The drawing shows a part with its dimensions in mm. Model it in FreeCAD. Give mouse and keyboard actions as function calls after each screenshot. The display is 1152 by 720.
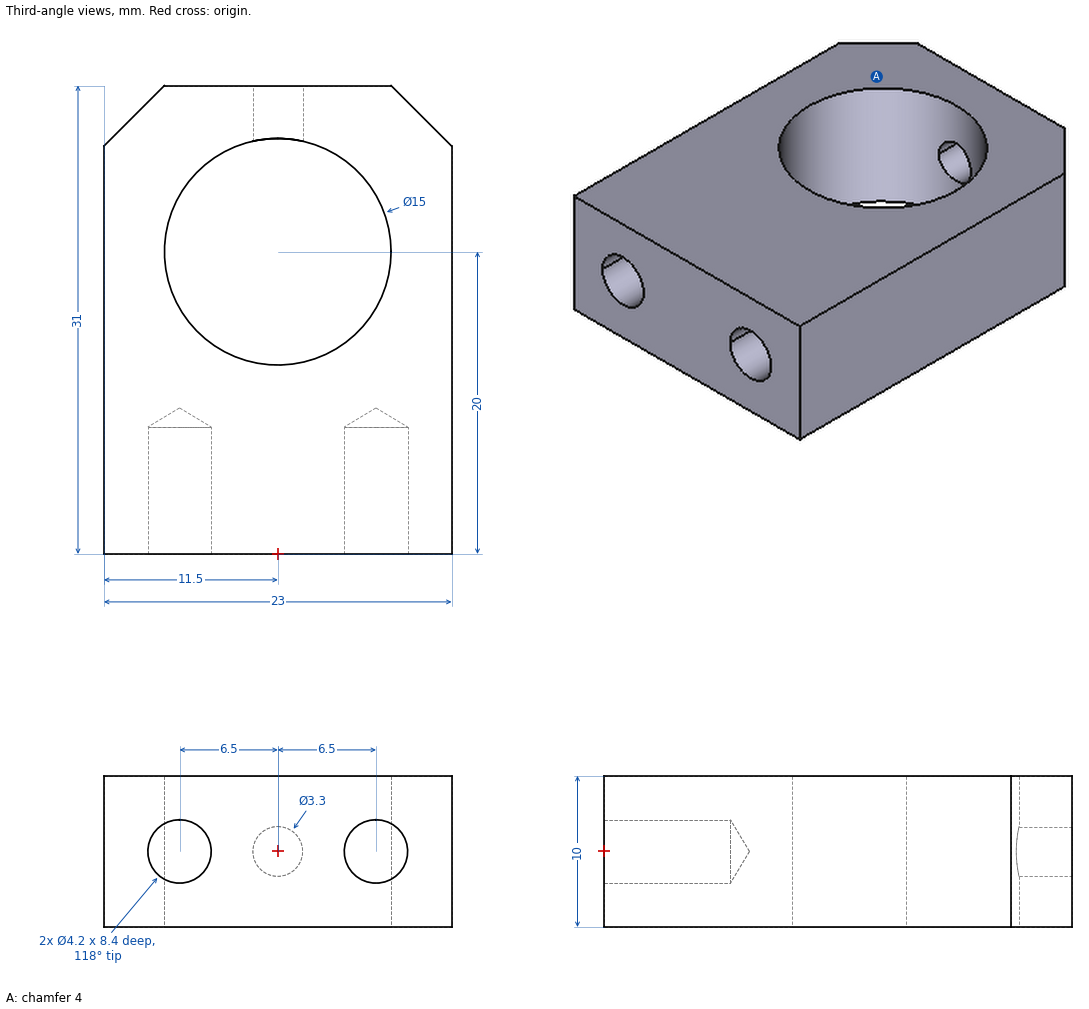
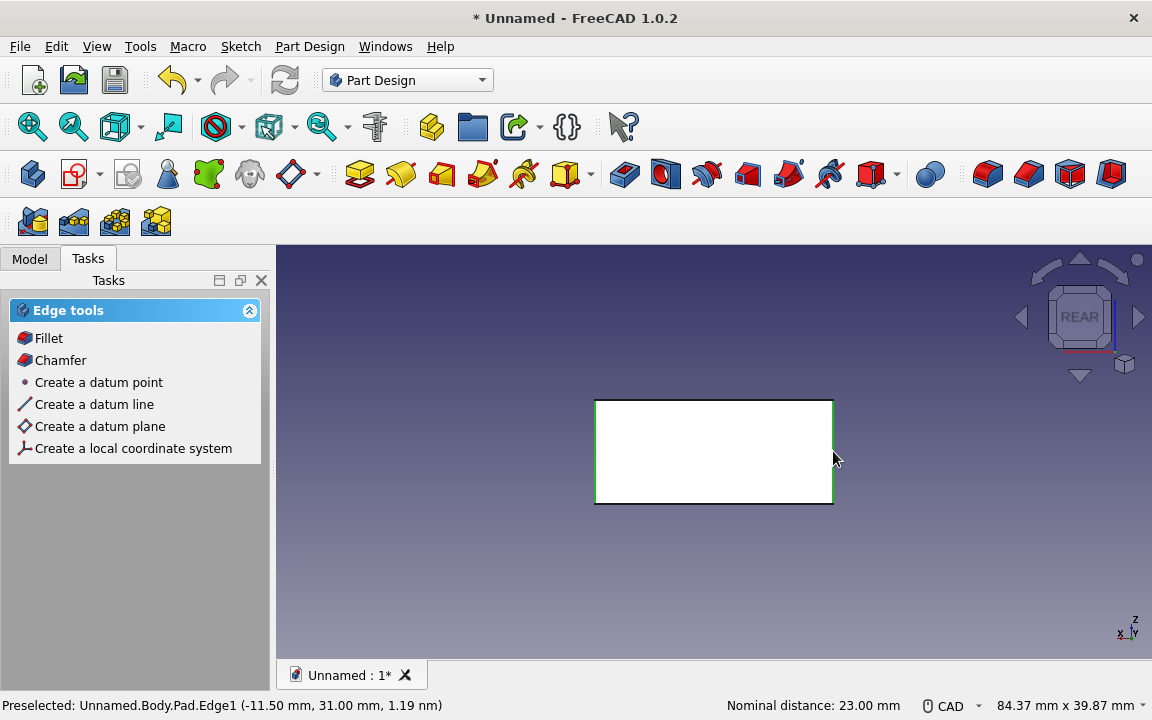
click(1029, 174)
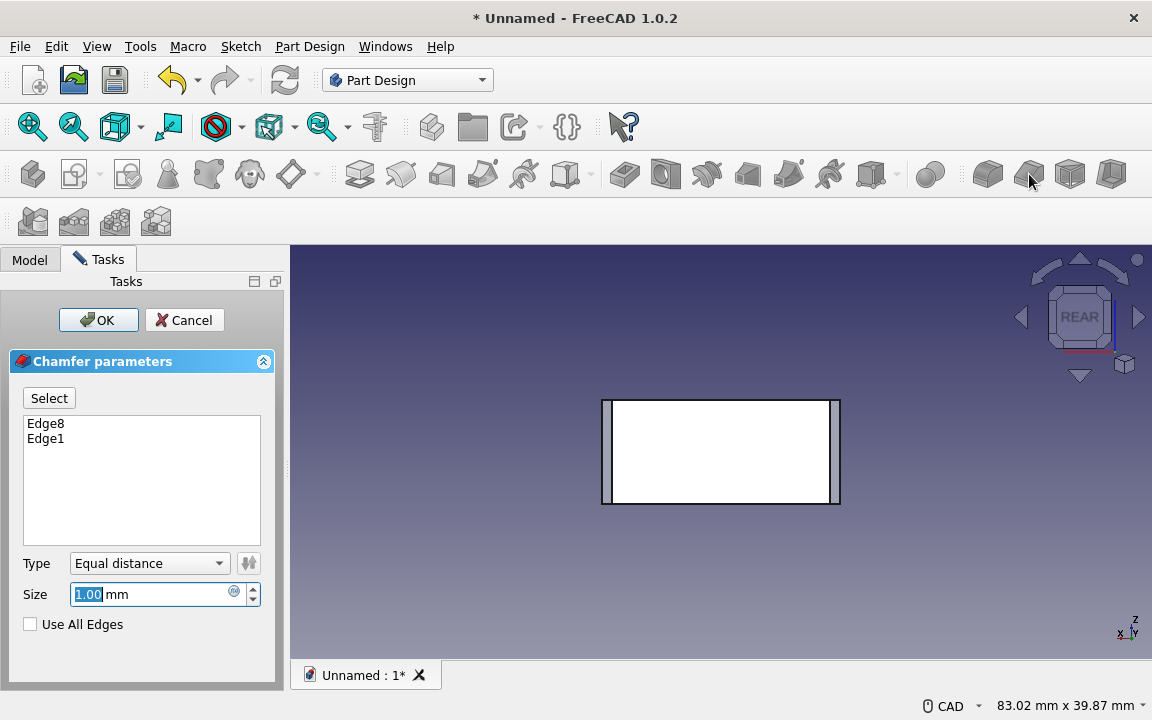
text(4)
key(Tab)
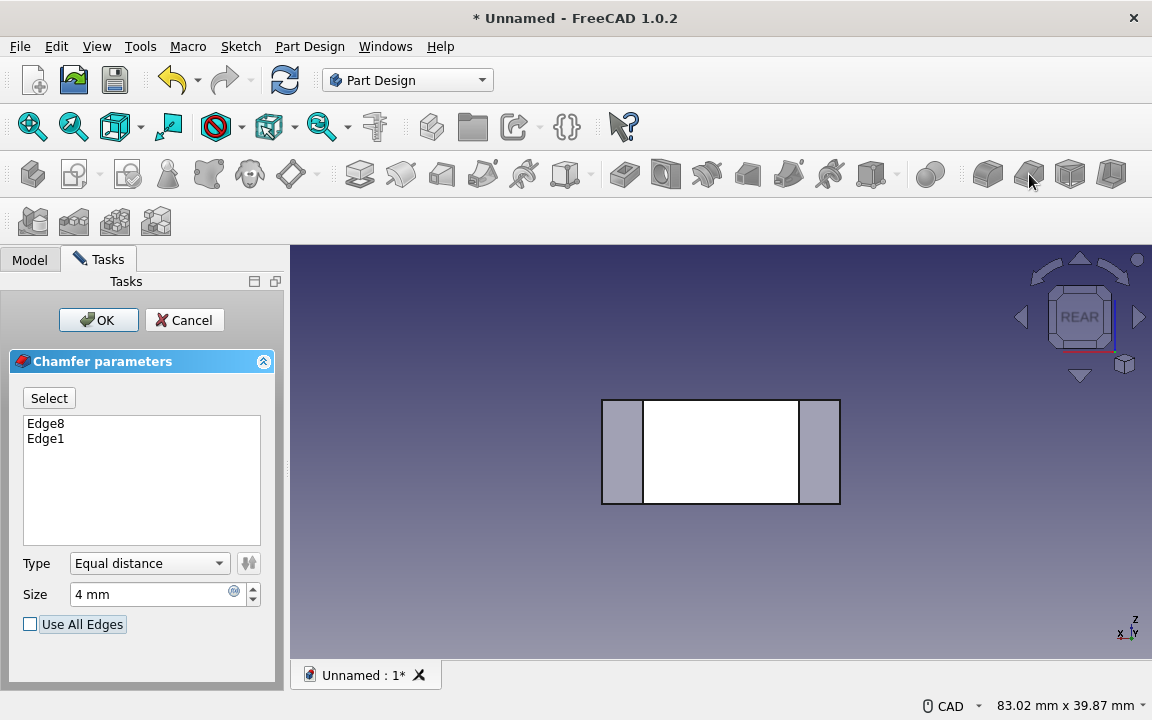
click(99, 320)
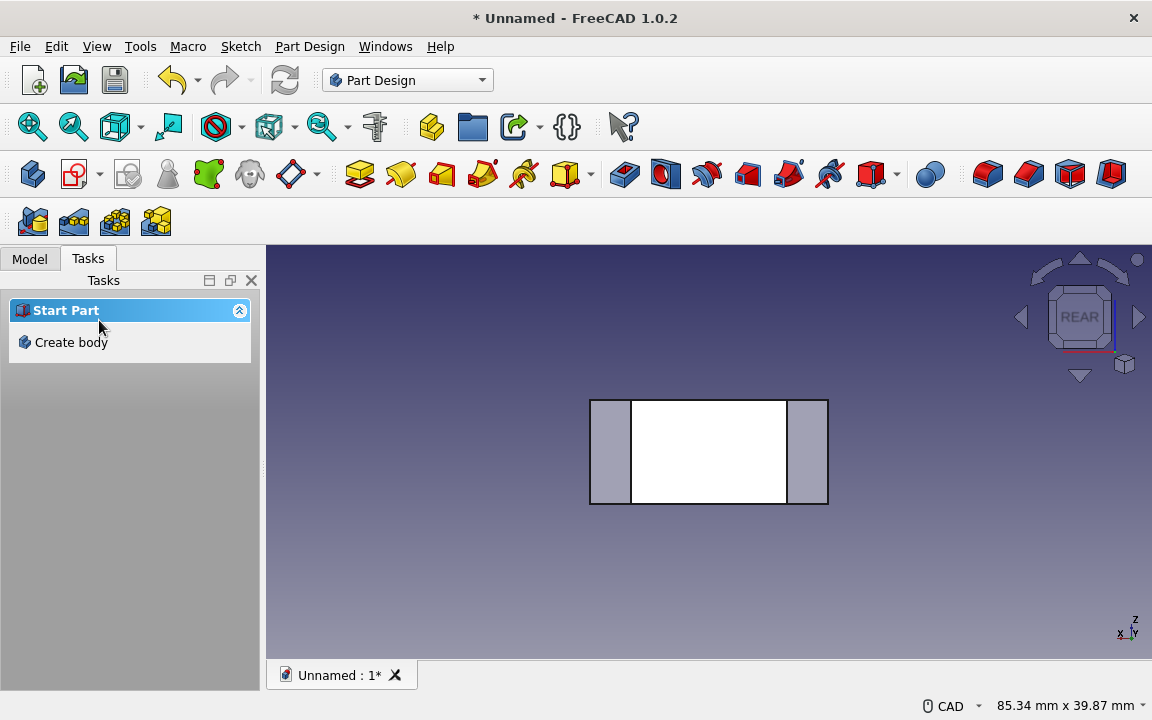
click(33, 128)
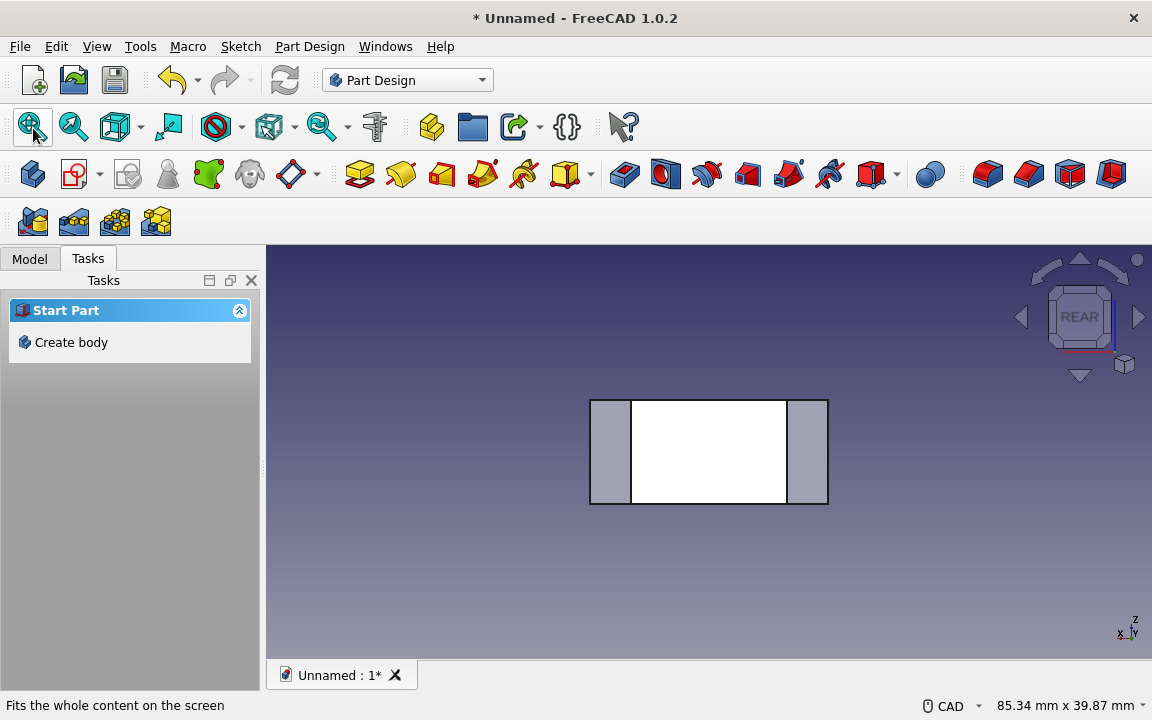
click(687, 451)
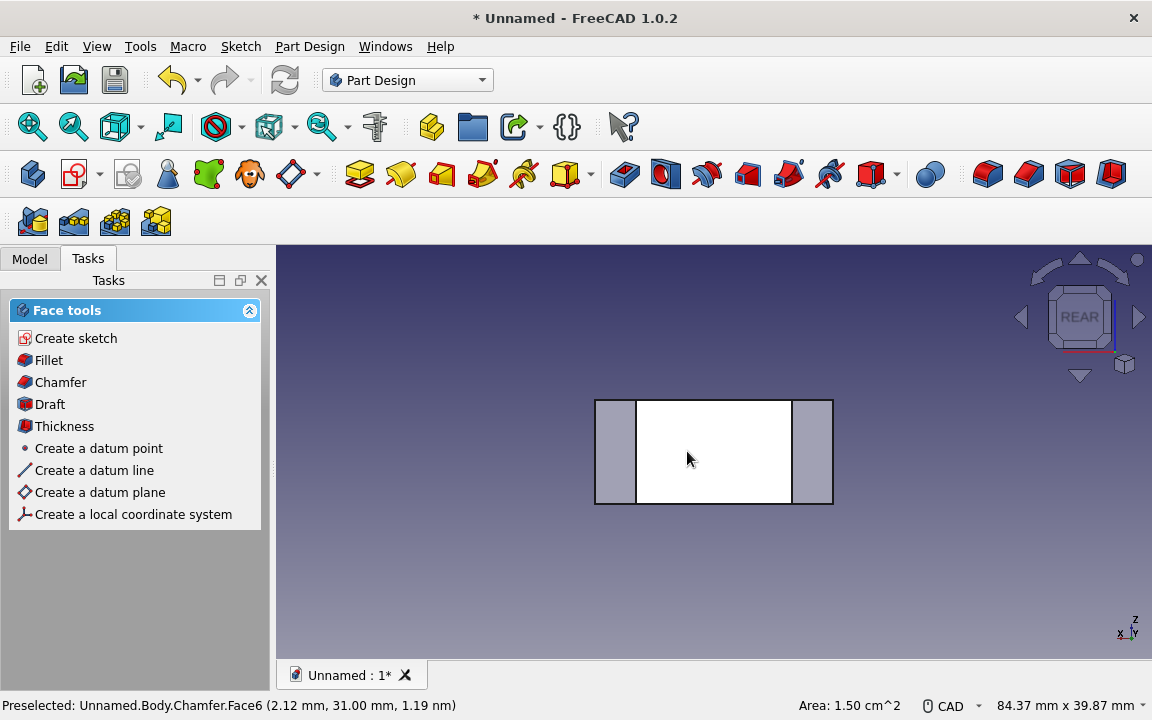
click(74, 174)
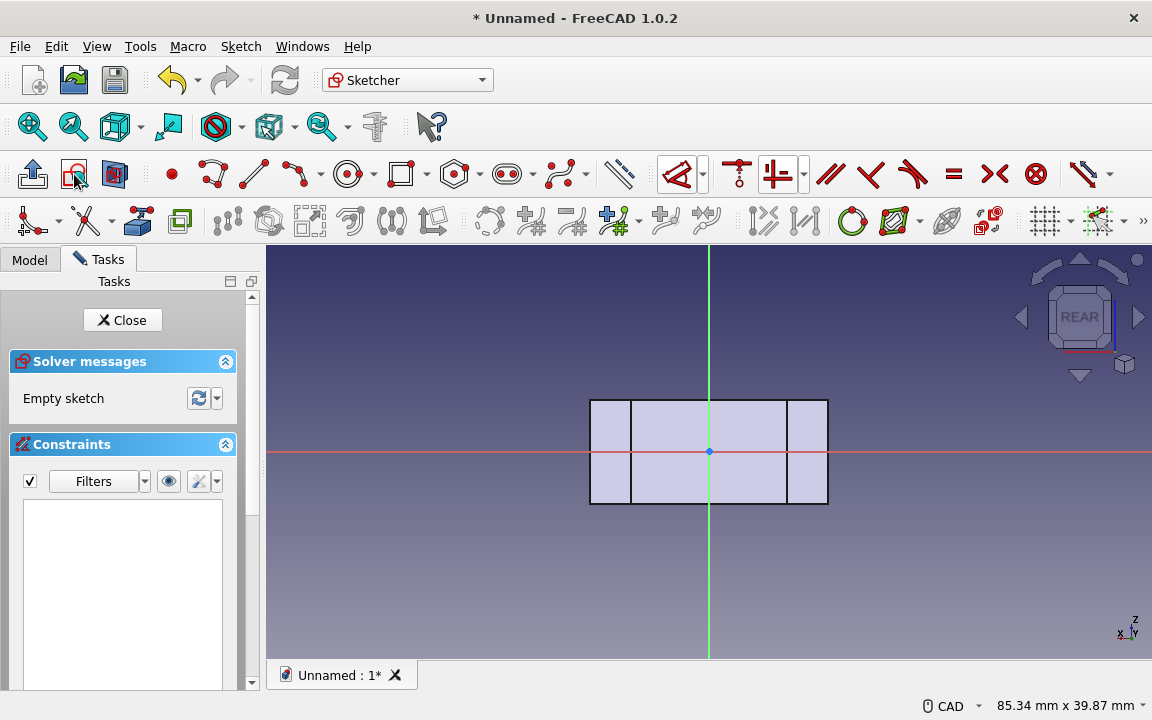
scroll(720, 452, up, 10)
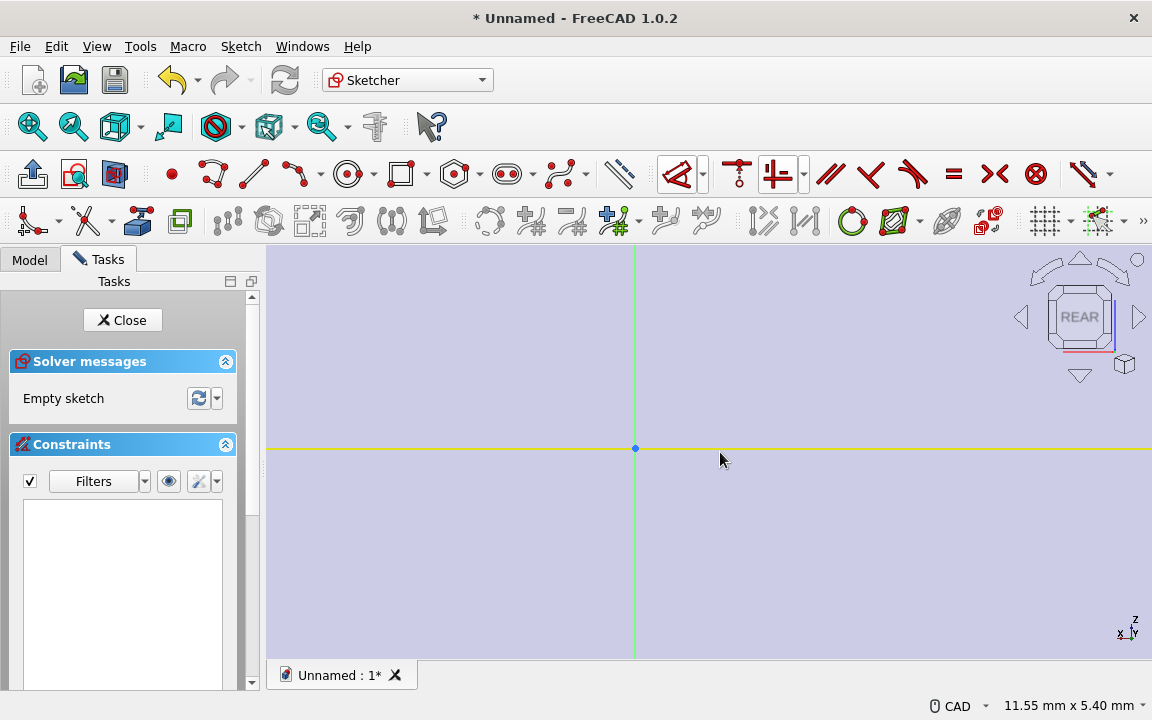
key(g)
key(c)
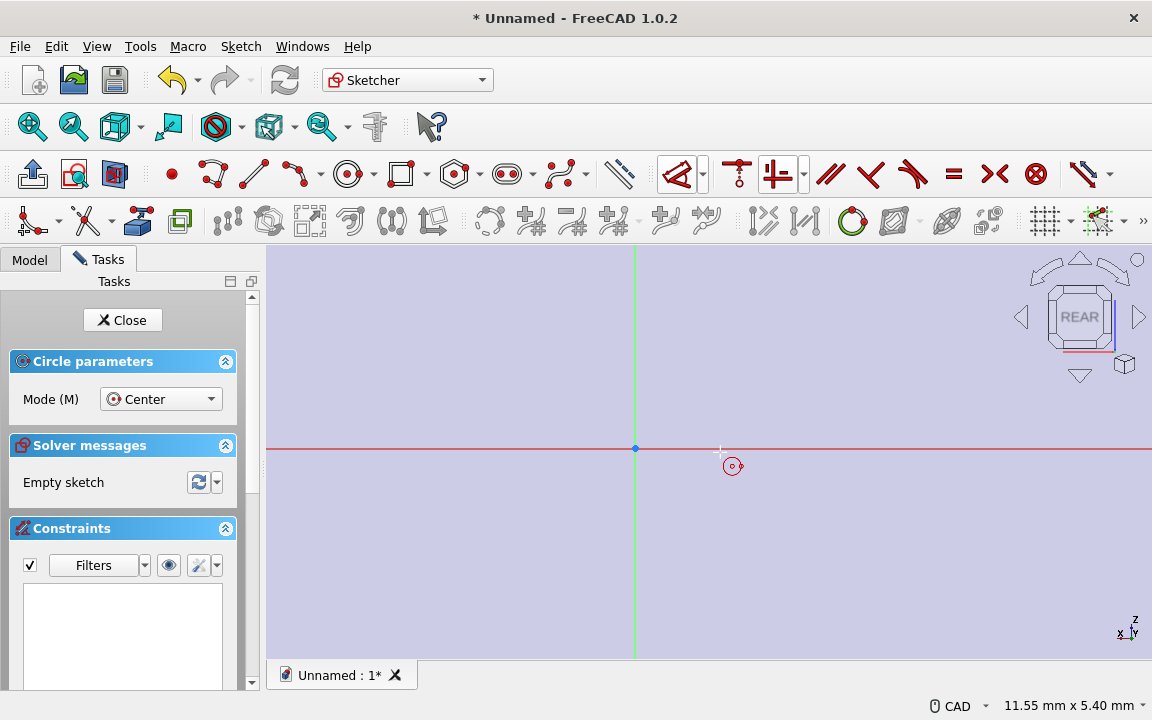
click(635, 449)
move(725, 359)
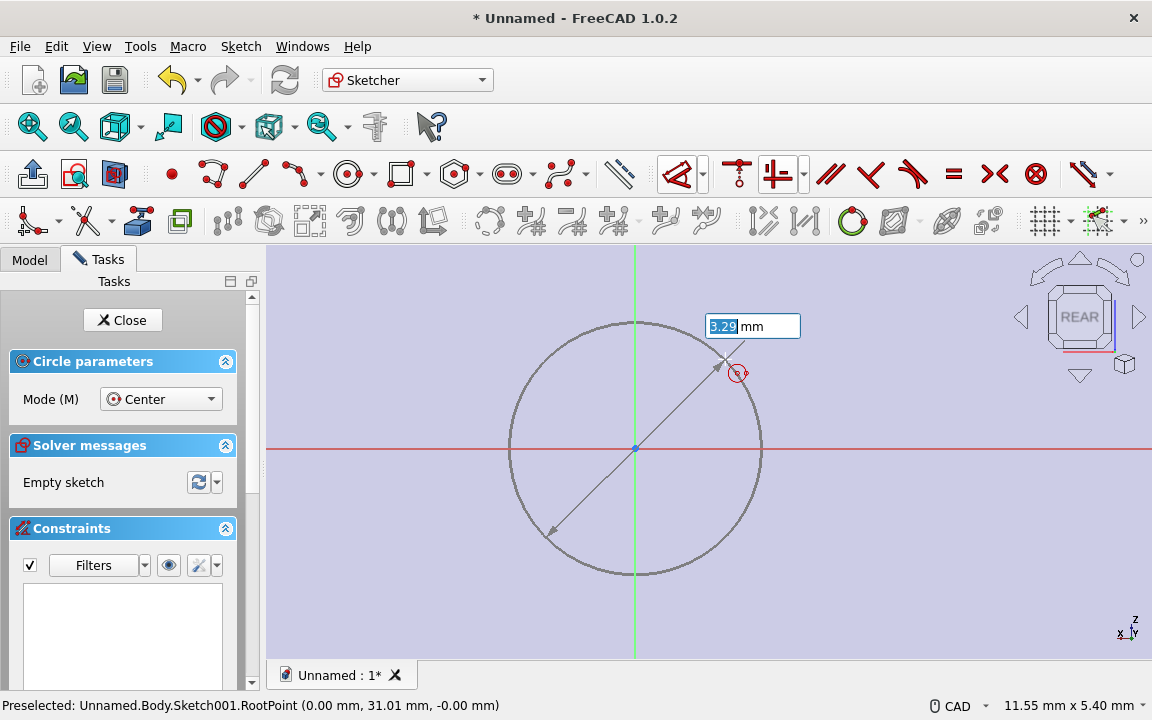
text(3.3)
key(Return)
key(Escape)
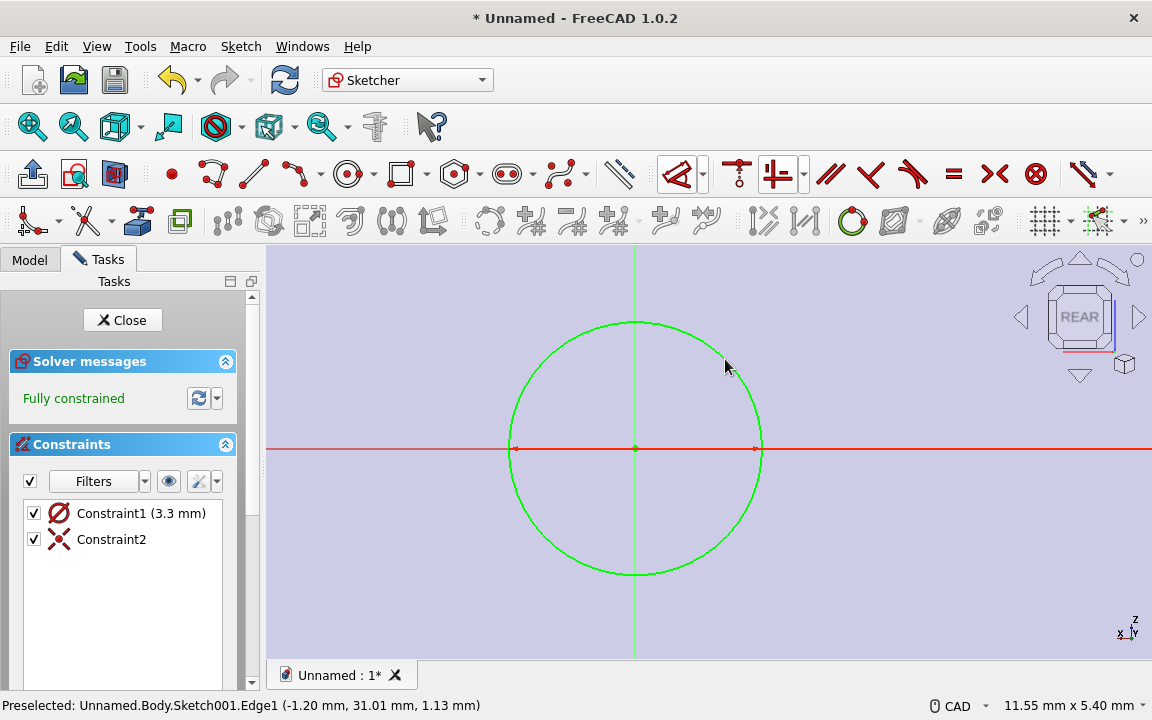
click(123, 320)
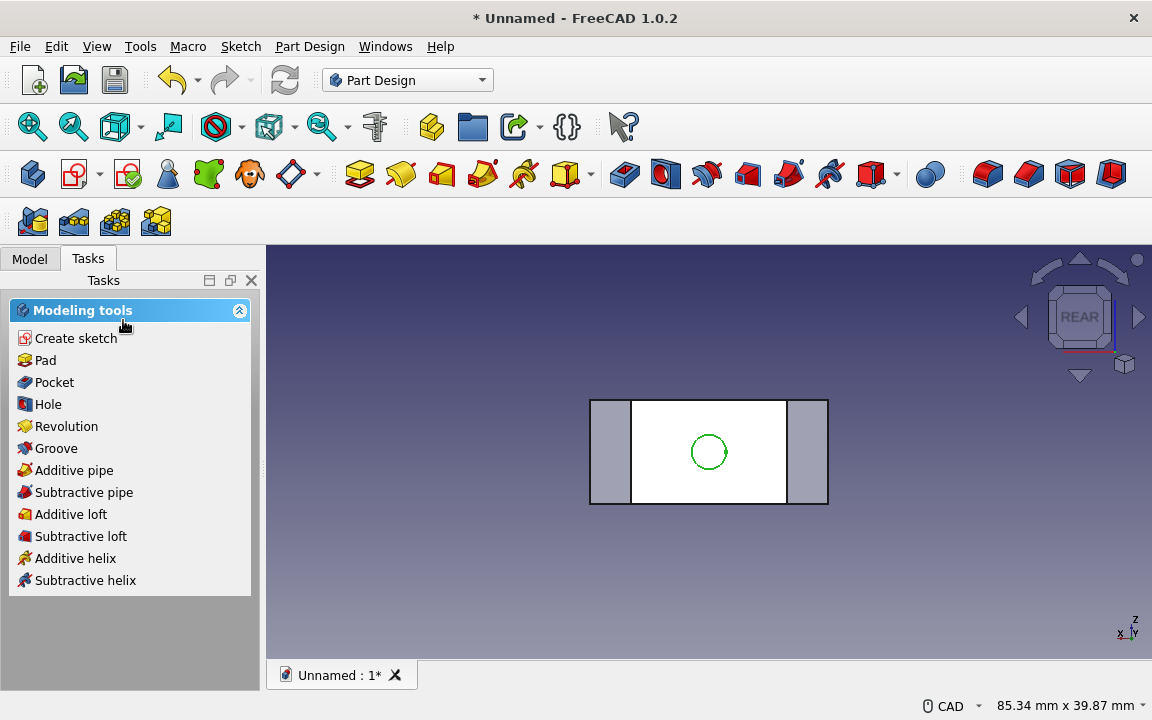
click(625, 174)